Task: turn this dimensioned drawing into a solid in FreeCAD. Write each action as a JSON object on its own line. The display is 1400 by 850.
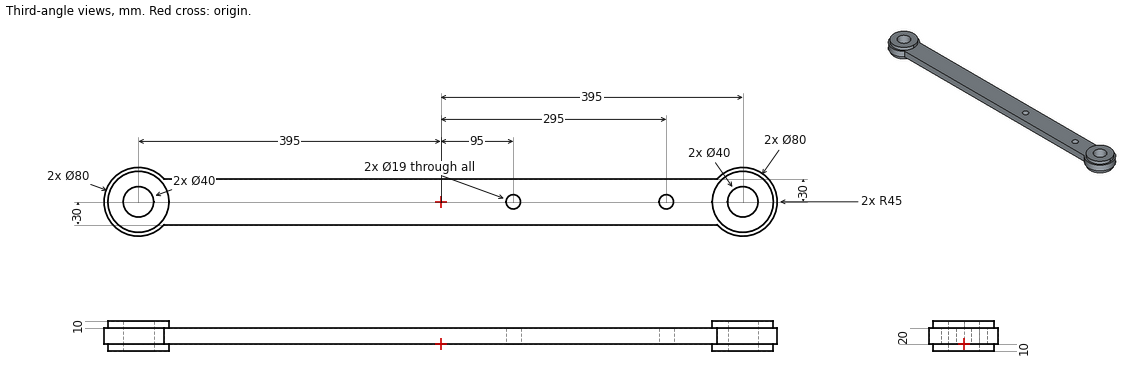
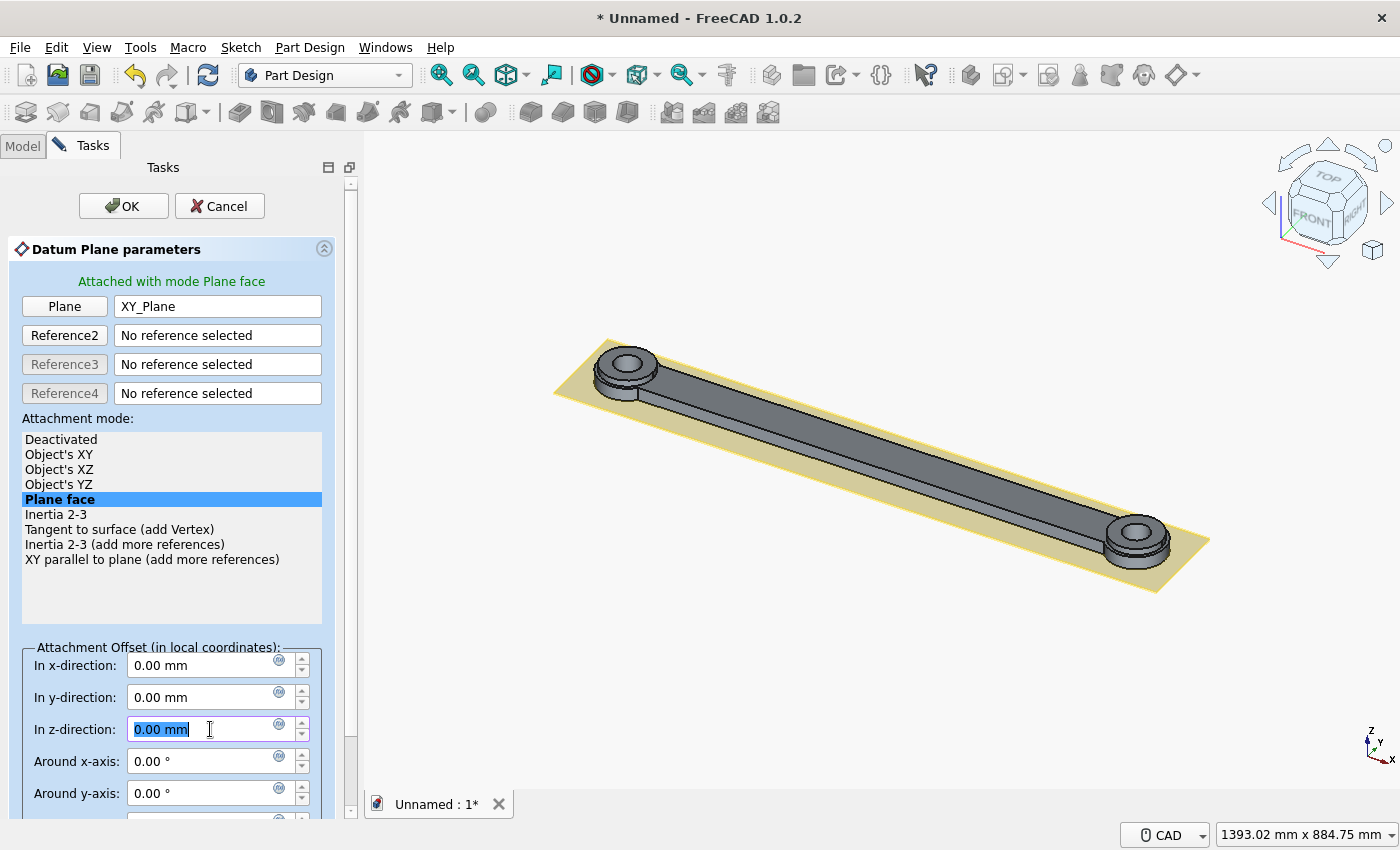
{"action": "type", "text": "-10"}
{"action": "key", "text": "Tab"}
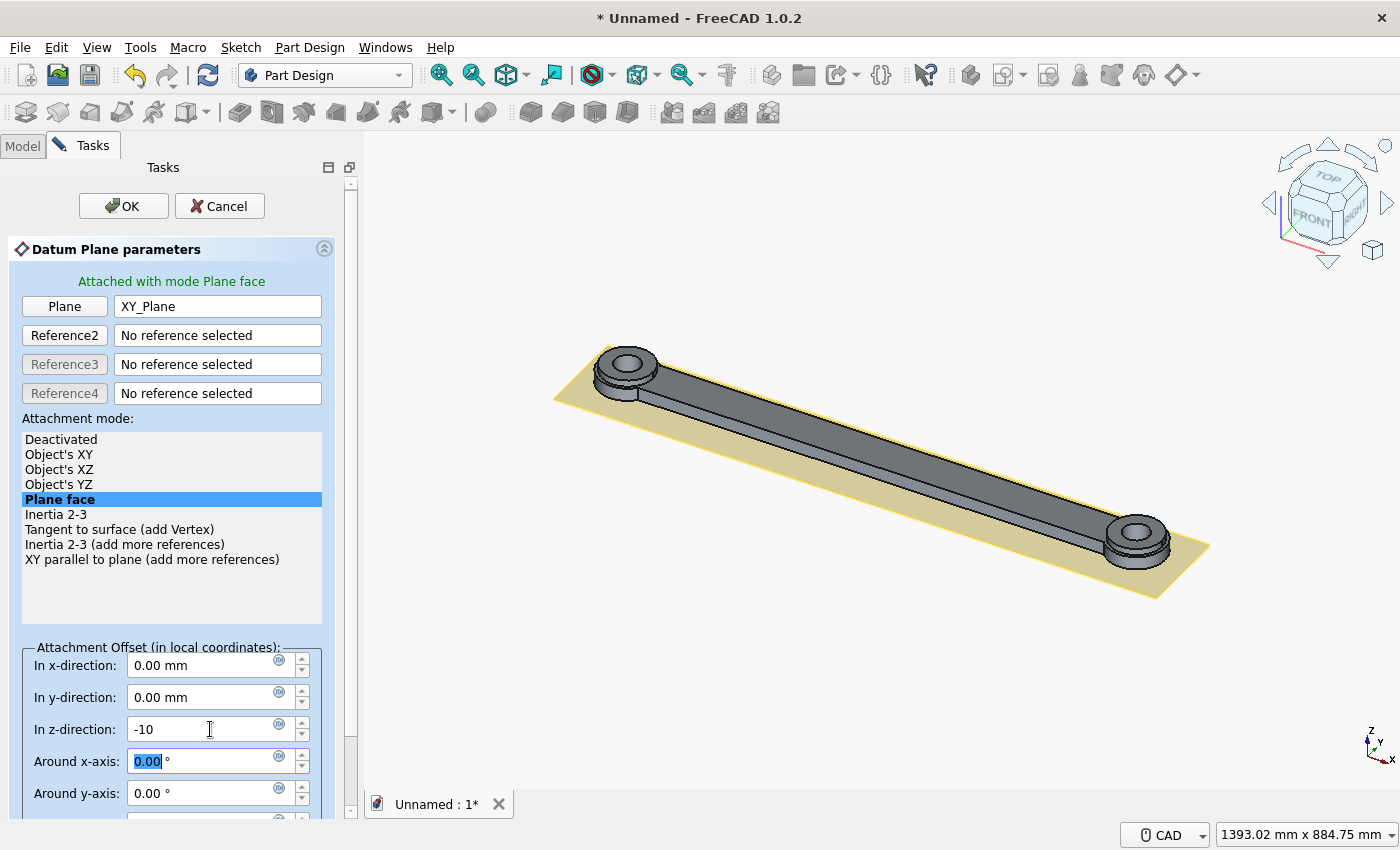
{"action": "left_click", "coordinate": [124, 206]}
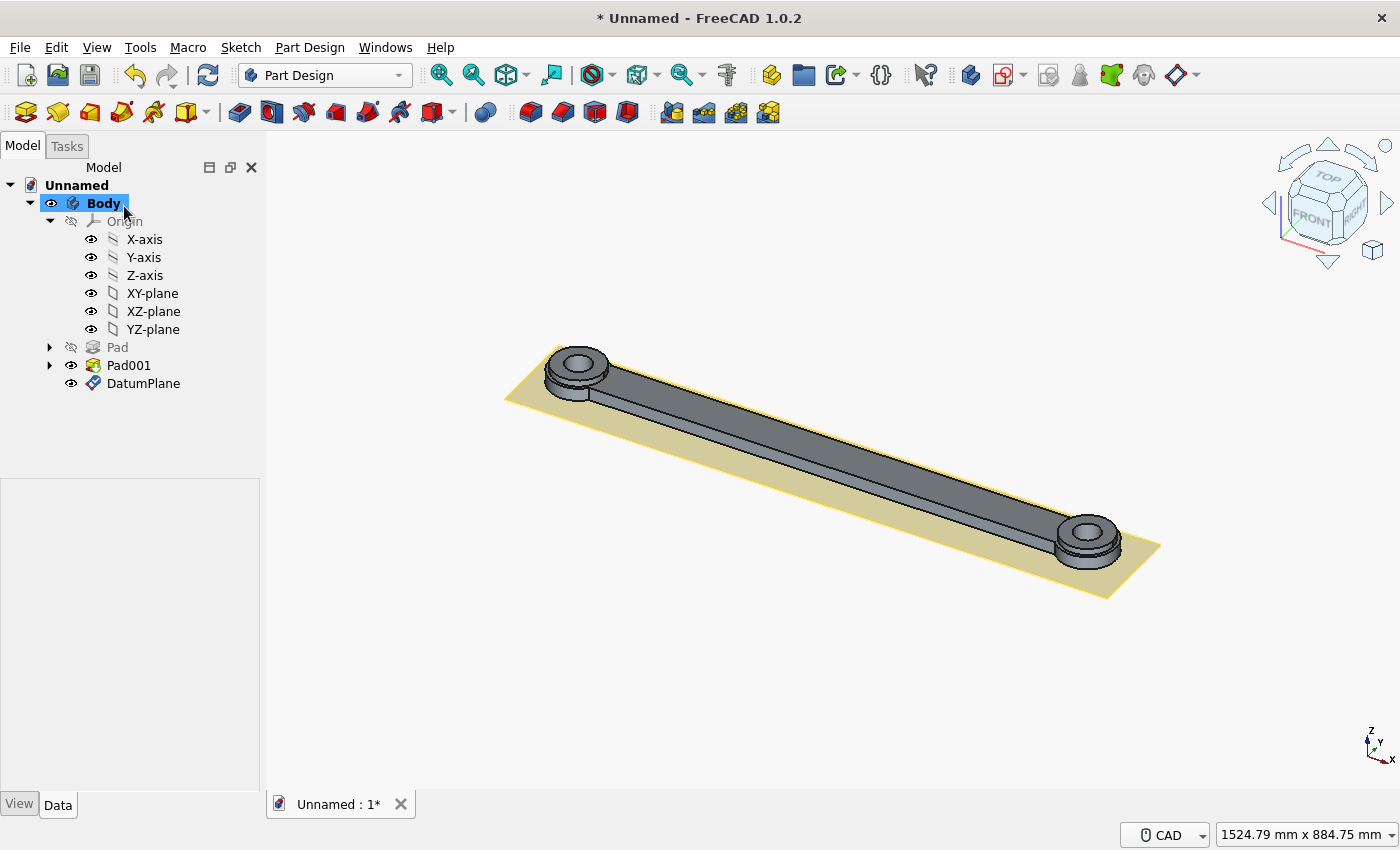
{"action": "left_click", "coordinate": [116, 383]}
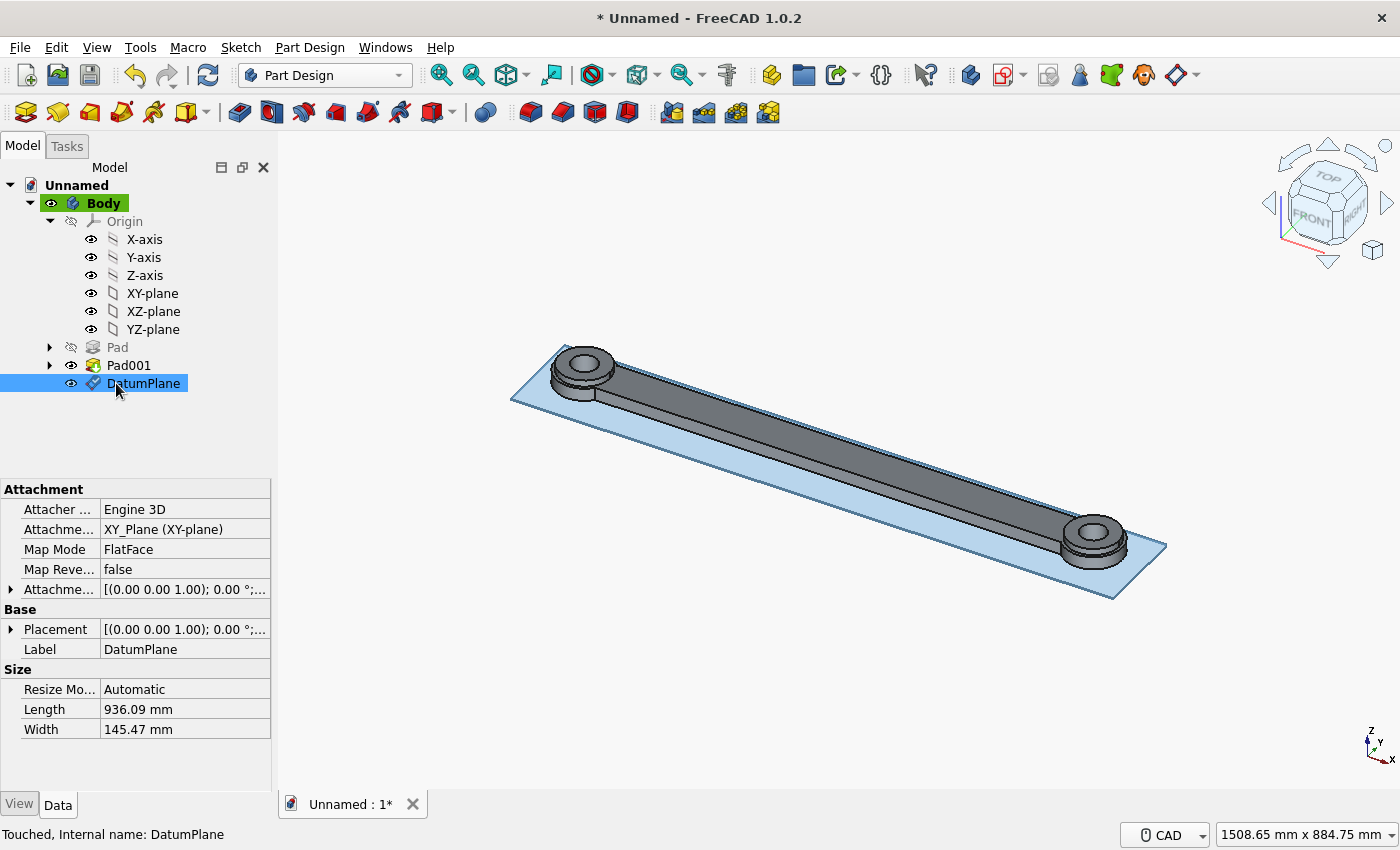
{"action": "left_click", "coordinate": [1004, 76]}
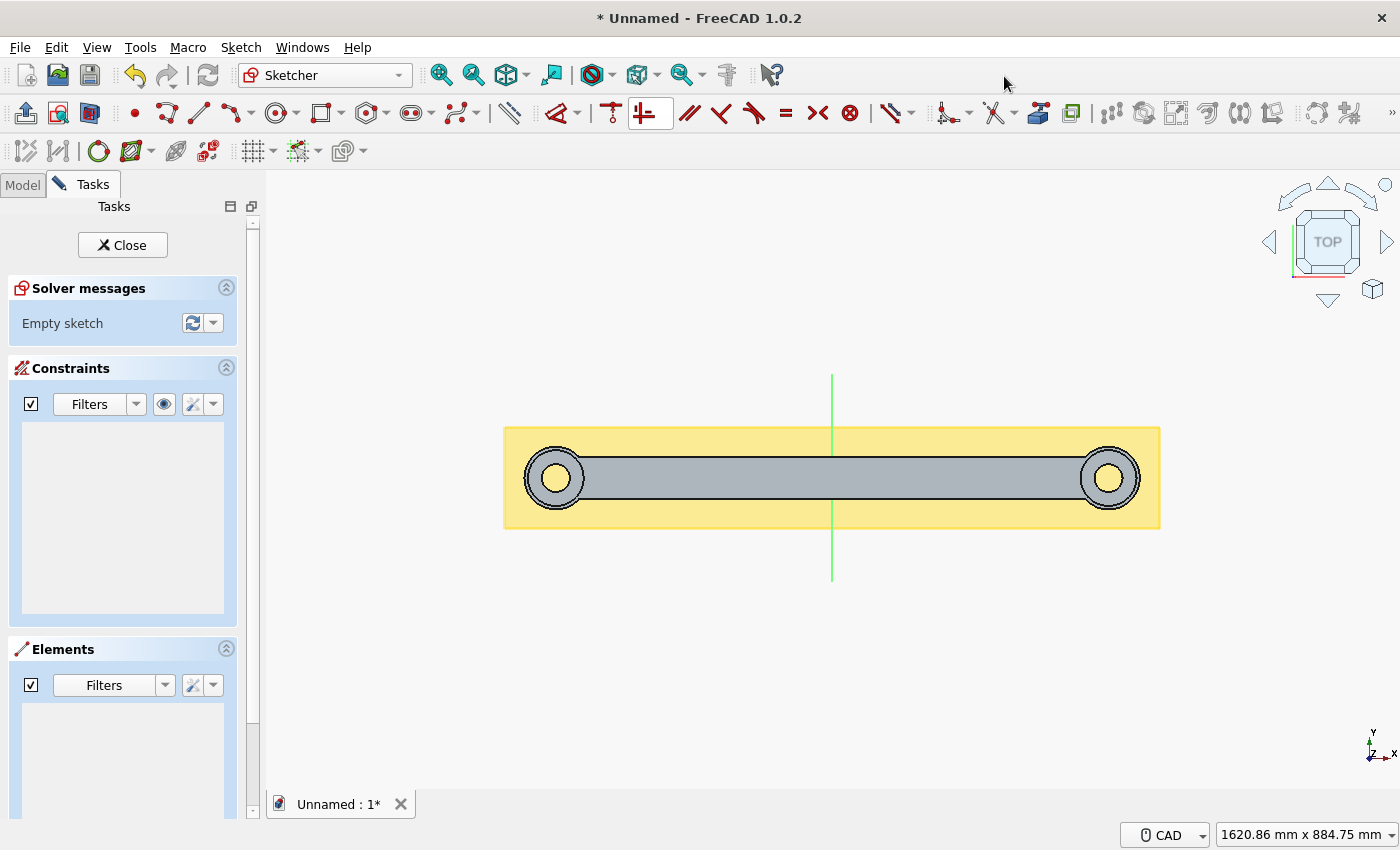
{"action": "left_click", "coordinate": [90, 114]}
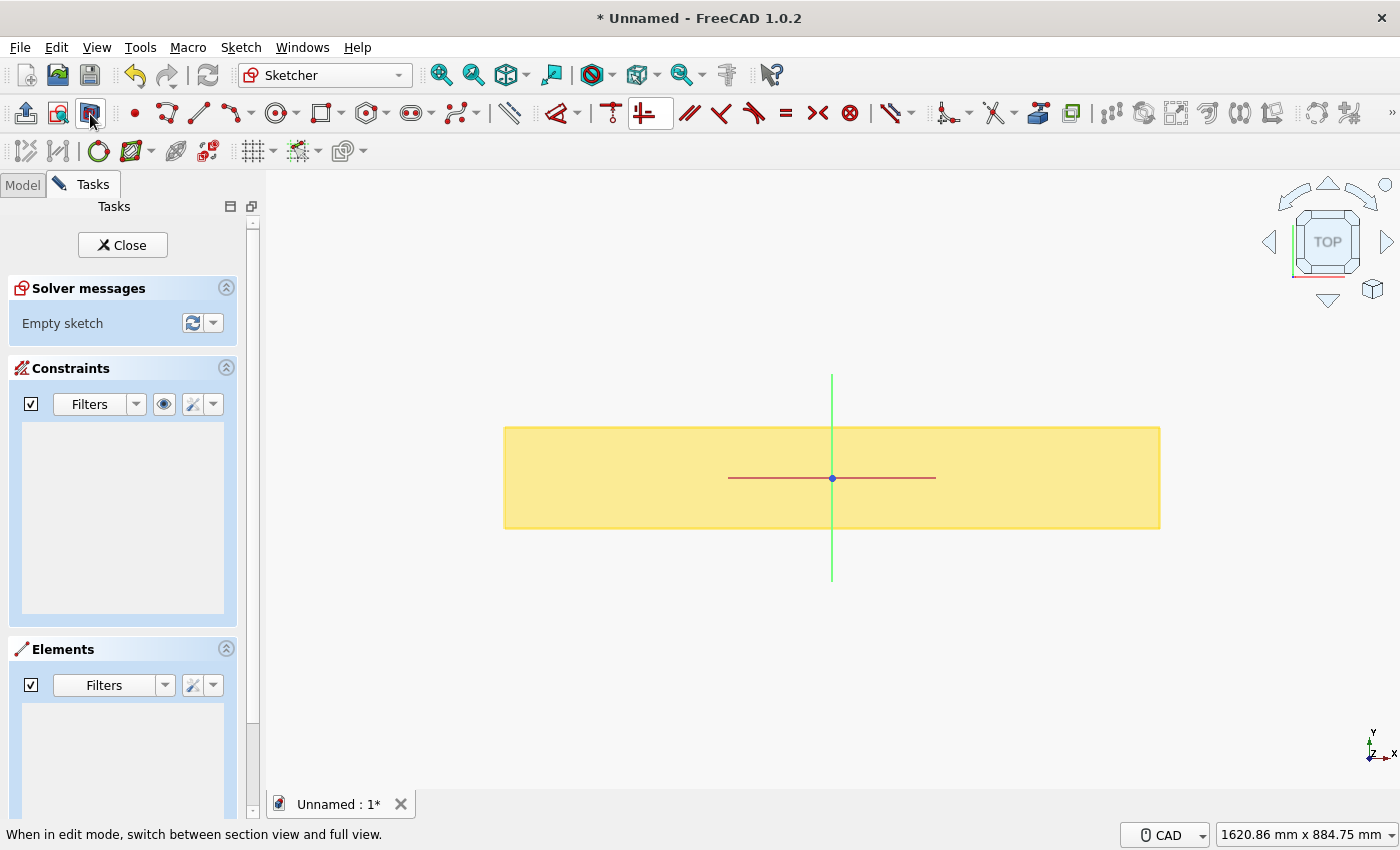
{"action": "left_click", "coordinate": [276, 114]}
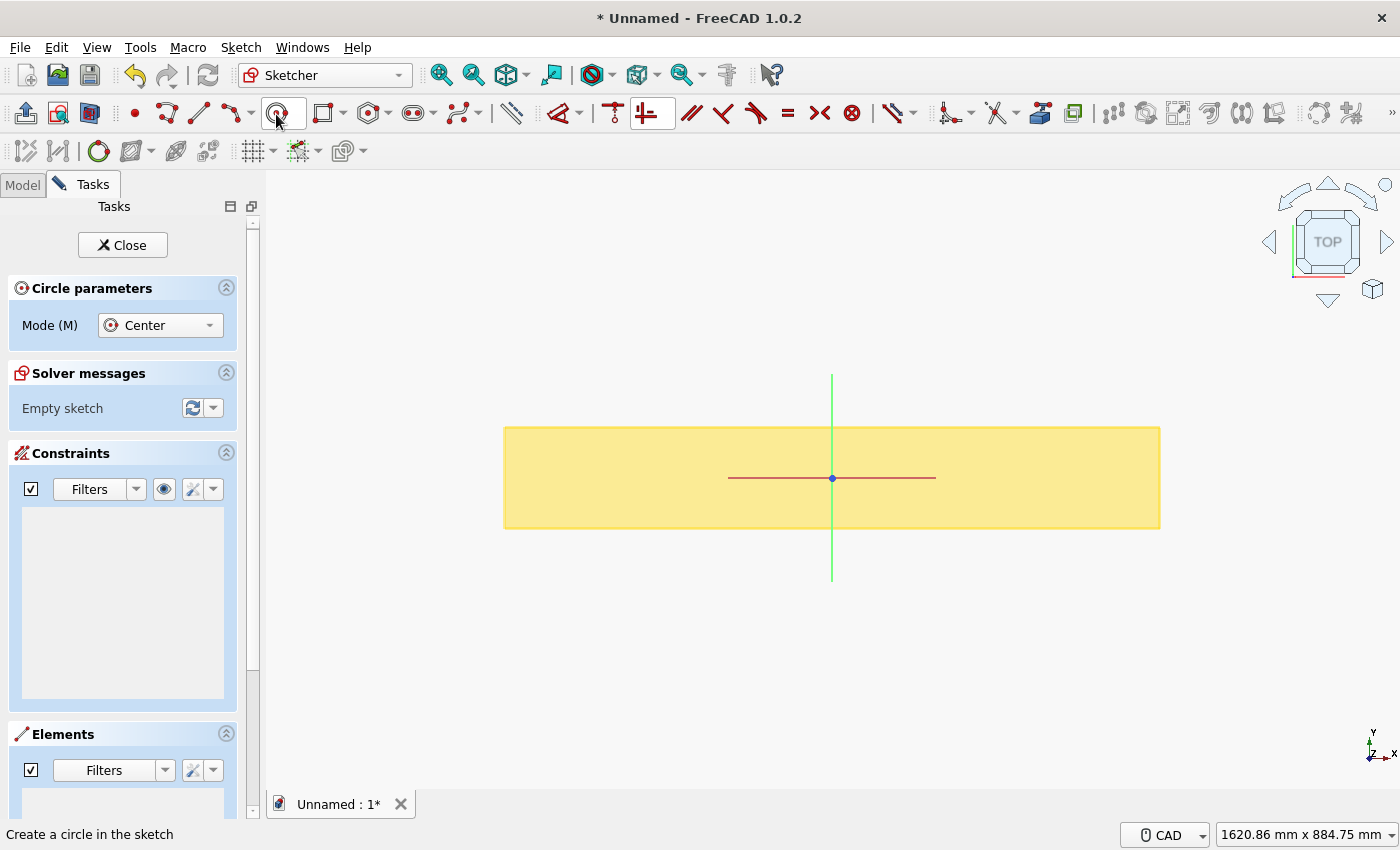
{"action": "left_click", "coordinate": [1109, 478]}
{"action": "left_click", "coordinate": [1128, 458]}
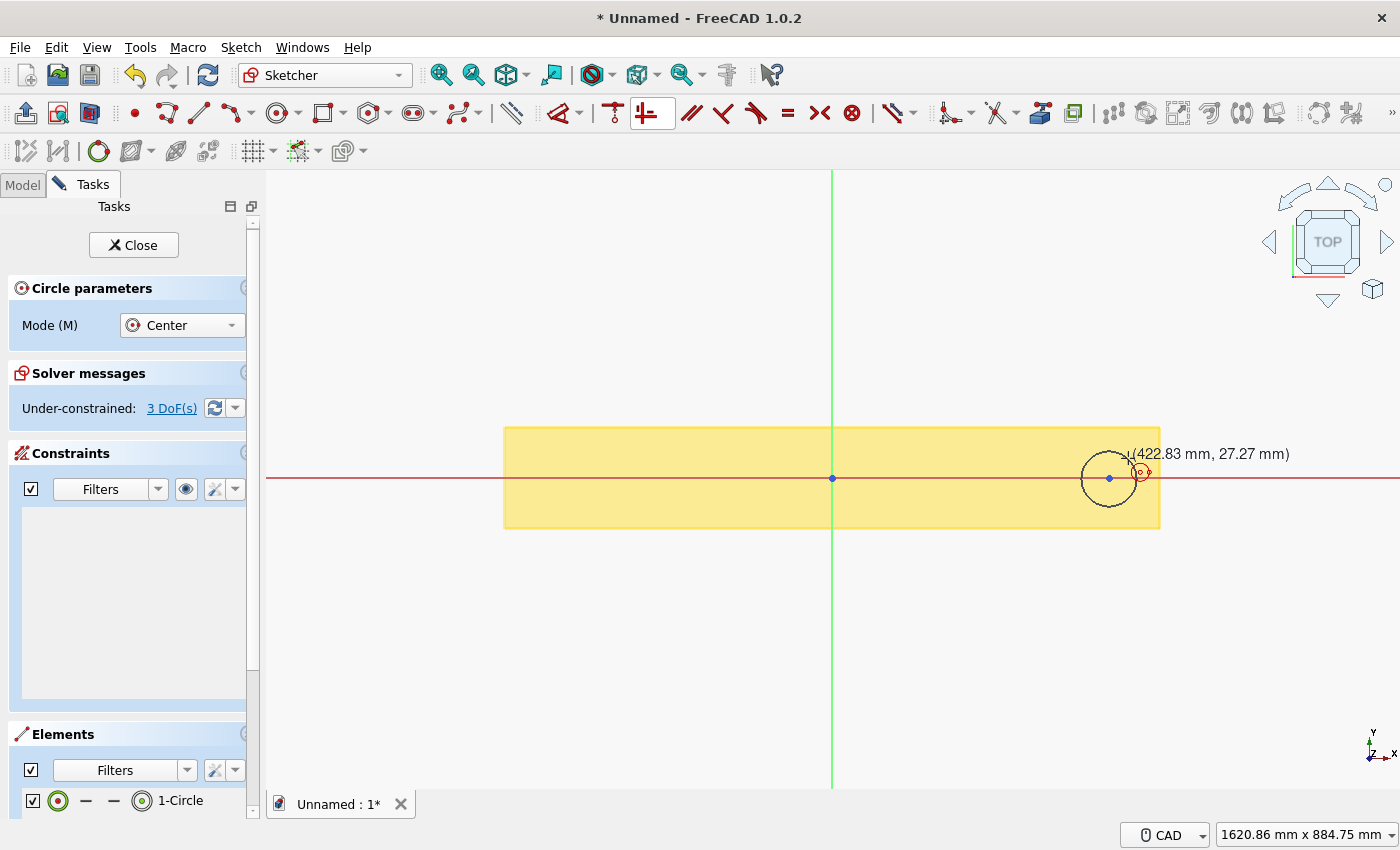
{"action": "left_click", "coordinate": [556, 478]}
{"action": "left_click", "coordinate": [576, 458]}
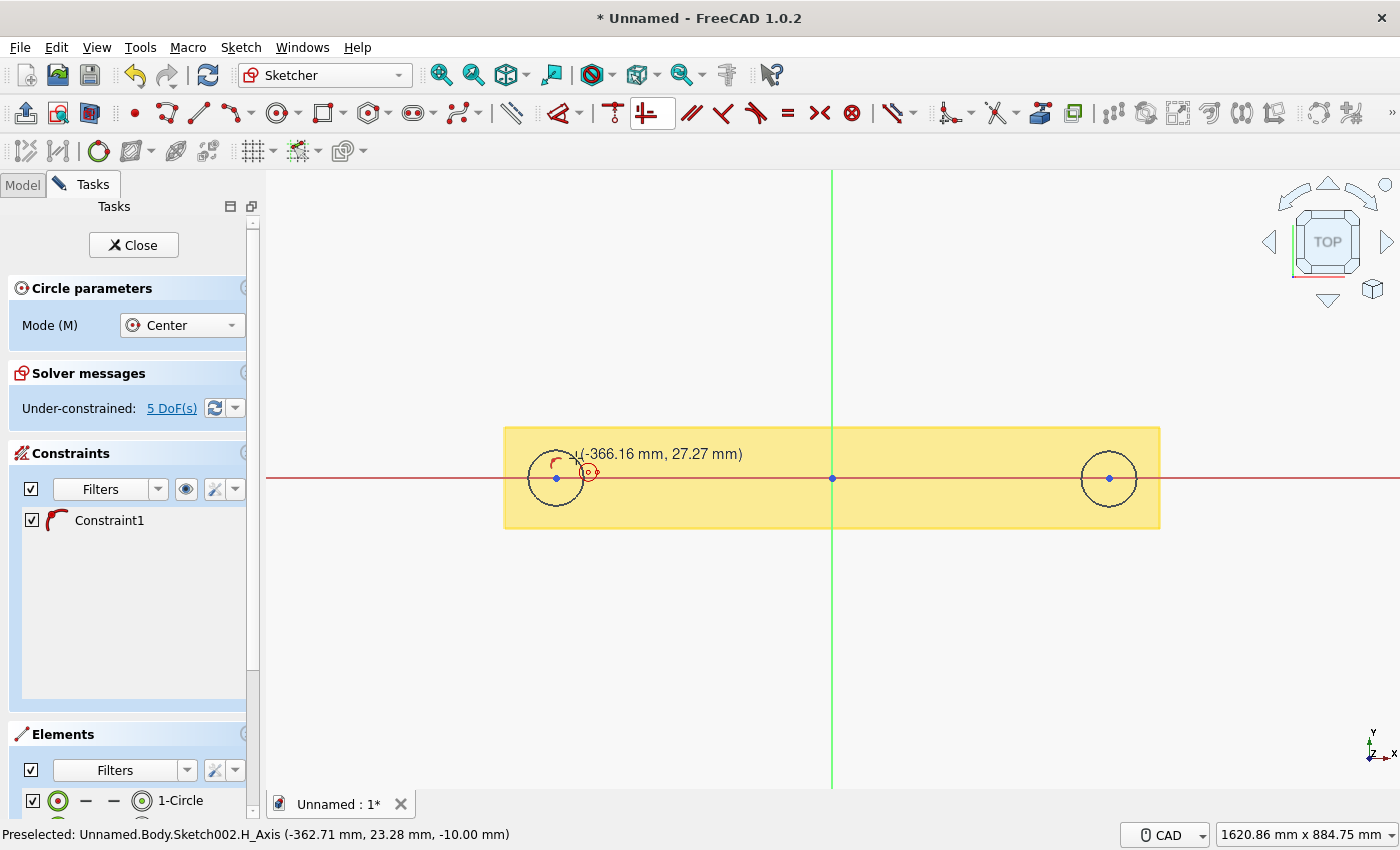
{"action": "scroll", "coordinate": [1109, 478], "scroll_direction": "up", "scroll_amount": 3}